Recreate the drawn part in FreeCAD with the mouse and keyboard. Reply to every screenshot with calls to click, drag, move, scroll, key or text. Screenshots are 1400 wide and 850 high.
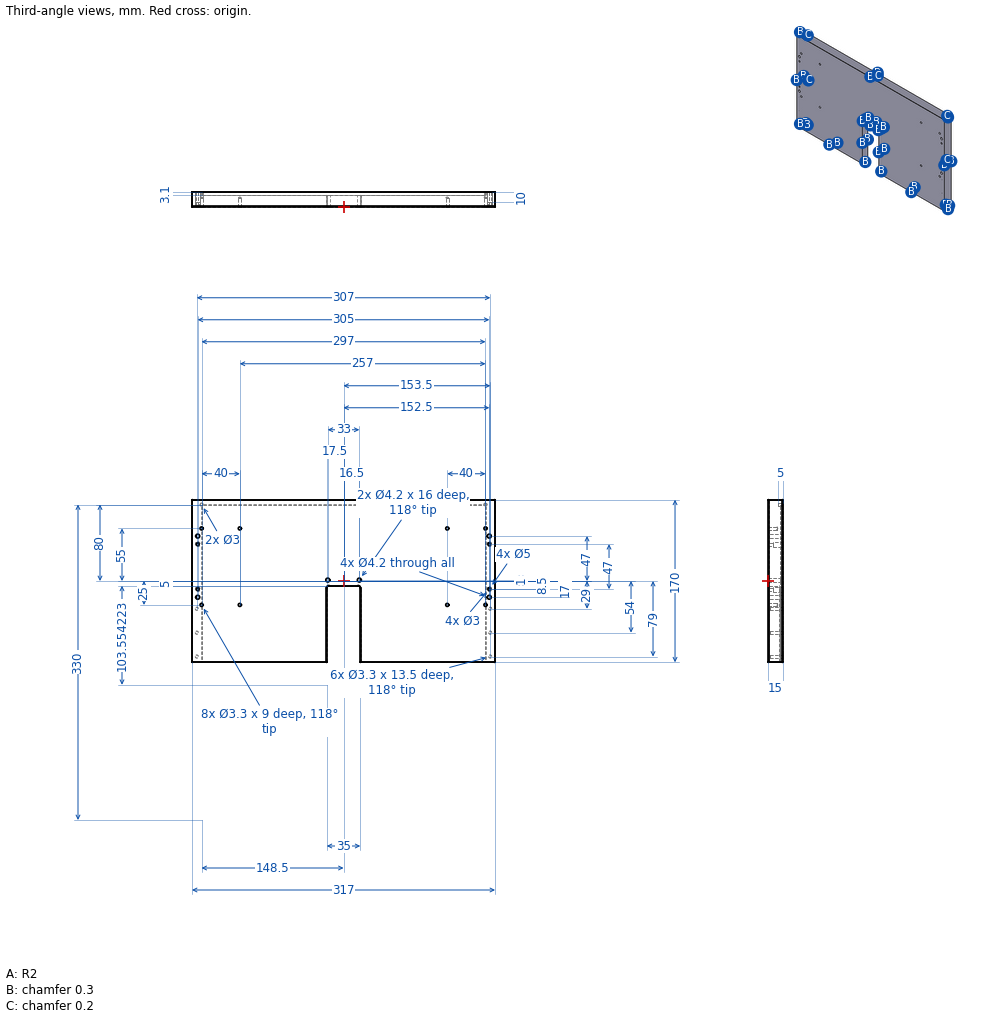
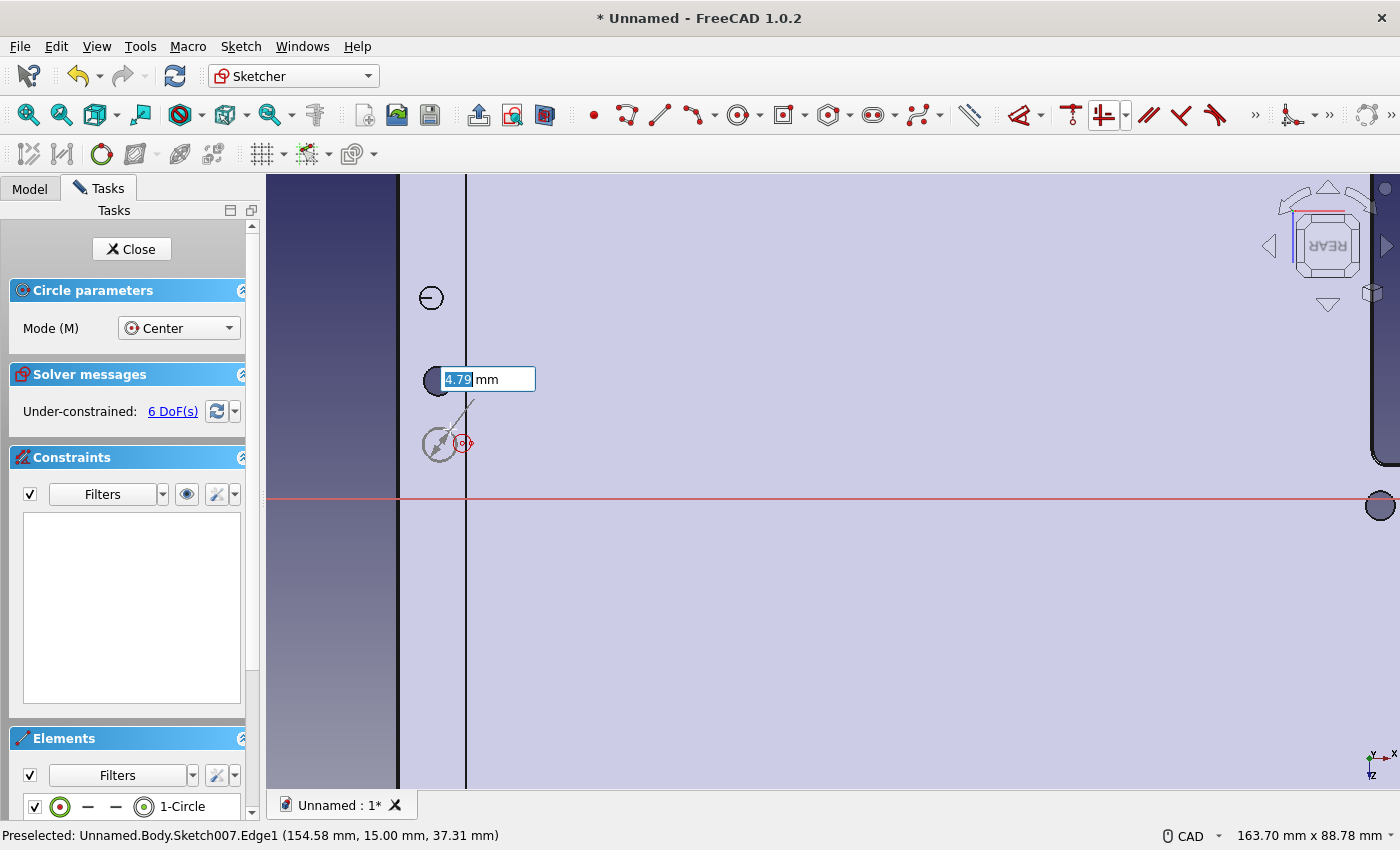
click(451, 428)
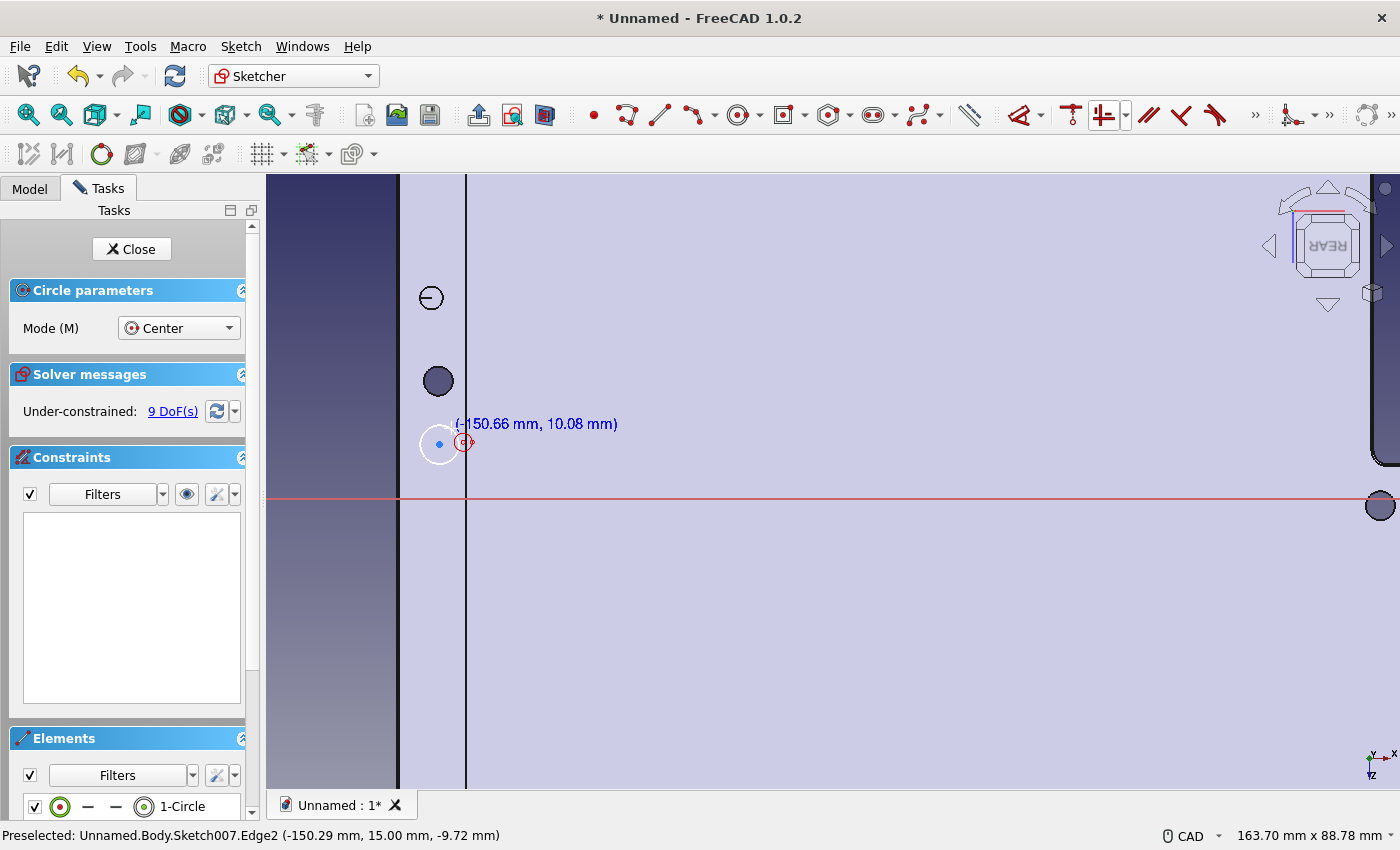
scroll(450, 429, down, 6)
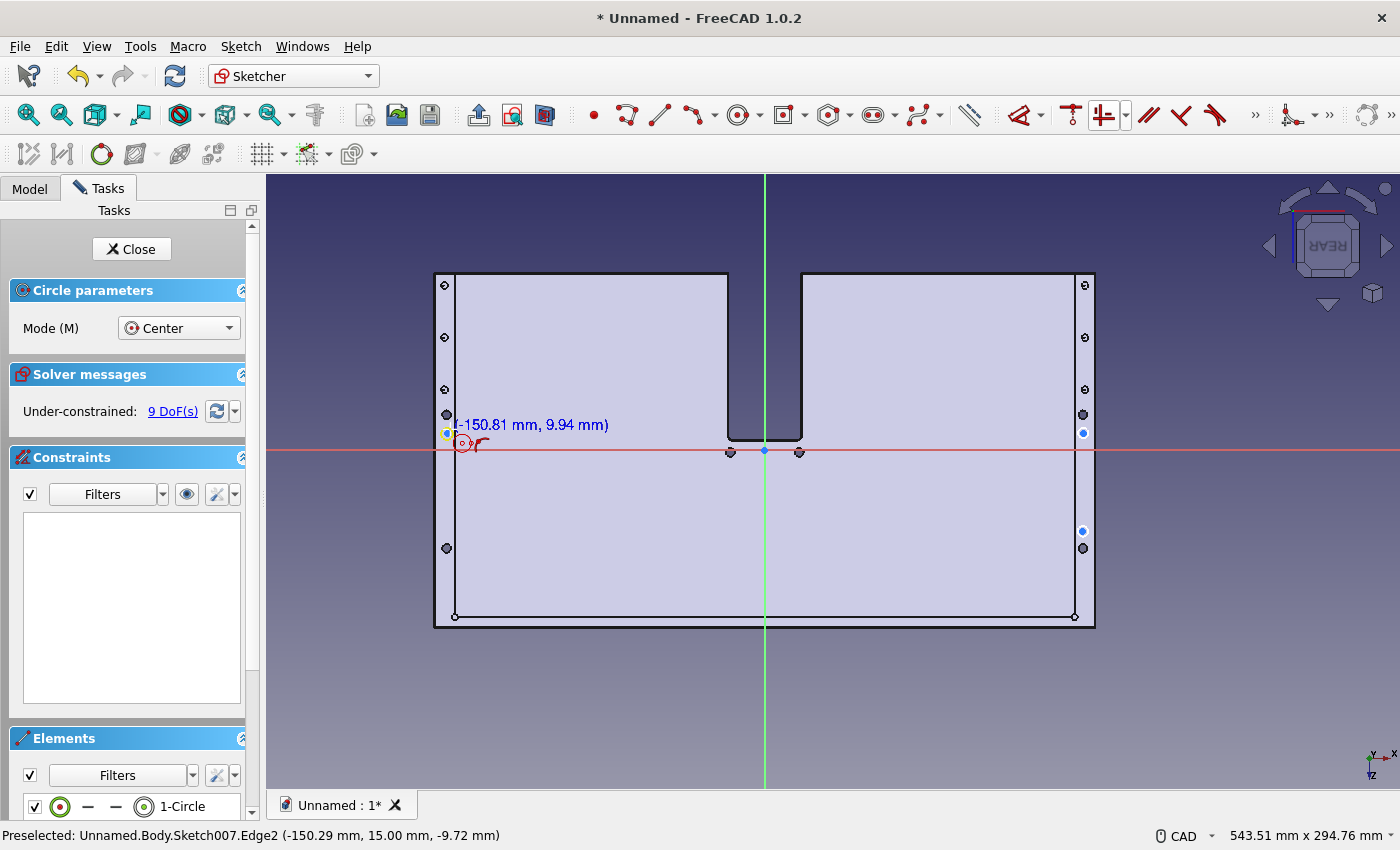
scroll(447, 531, up, 8)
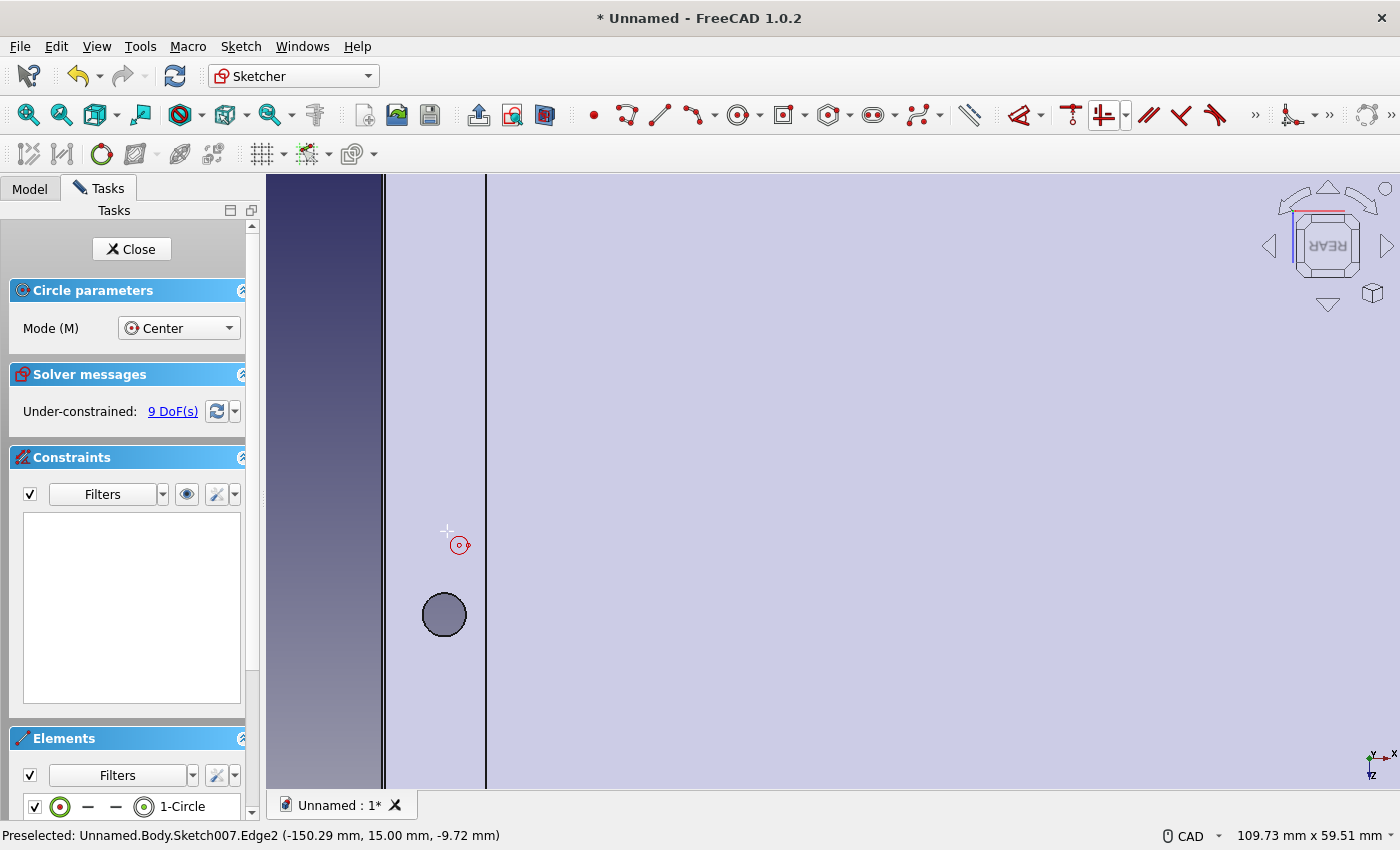
scroll(447, 531, down, 8)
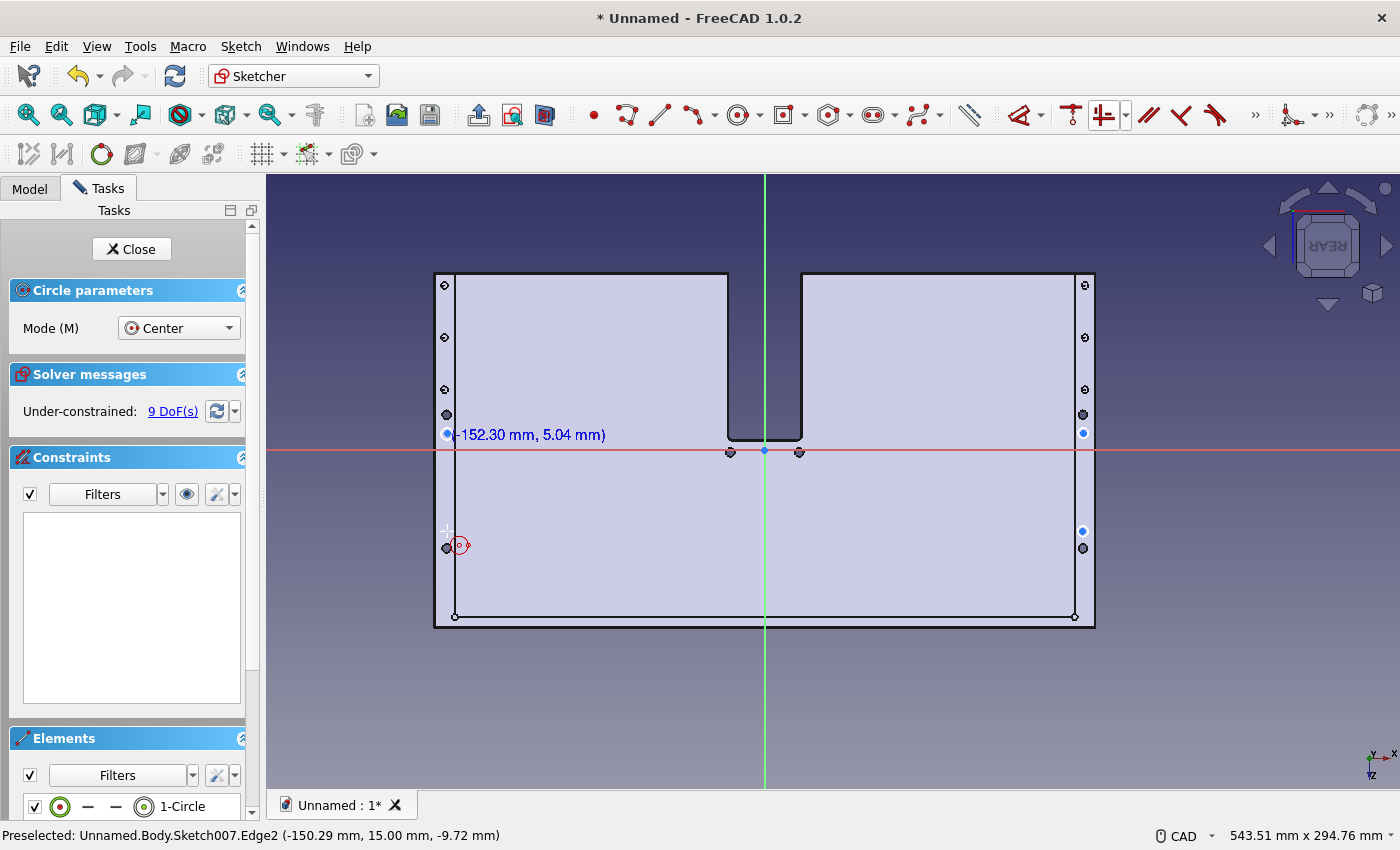
click(447, 531)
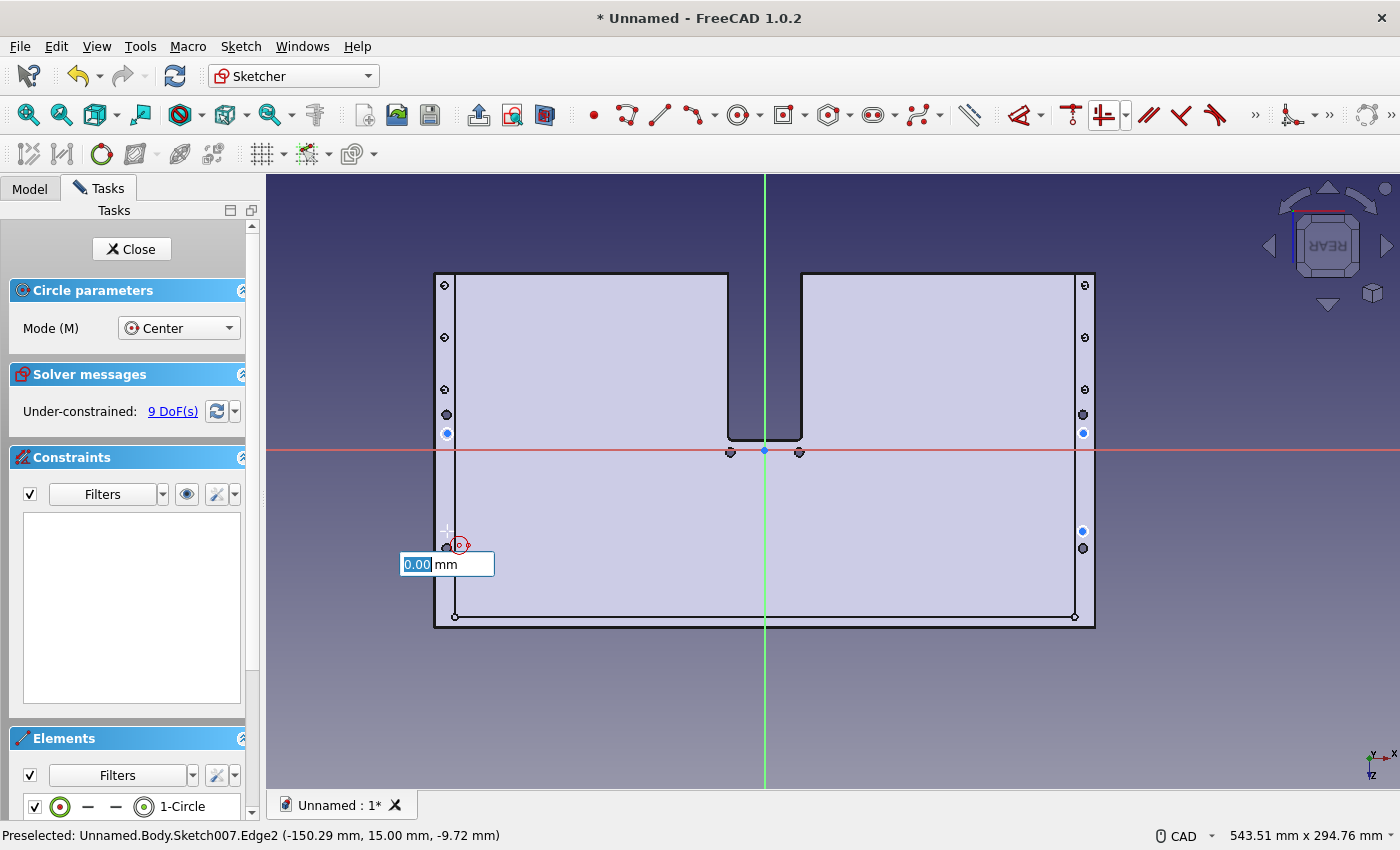
scroll(450, 527, up, 6)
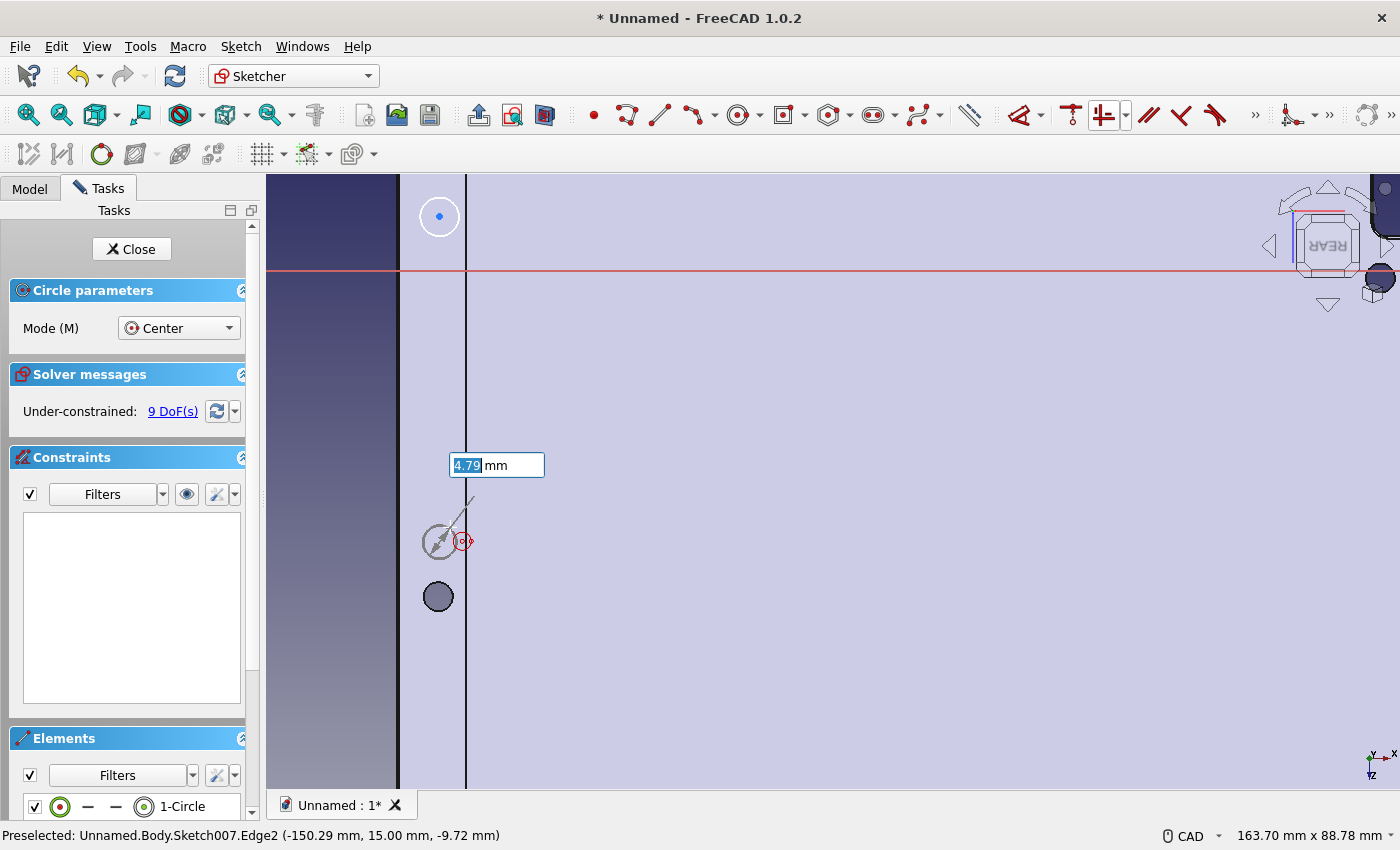
click(451, 526)
key(Escape)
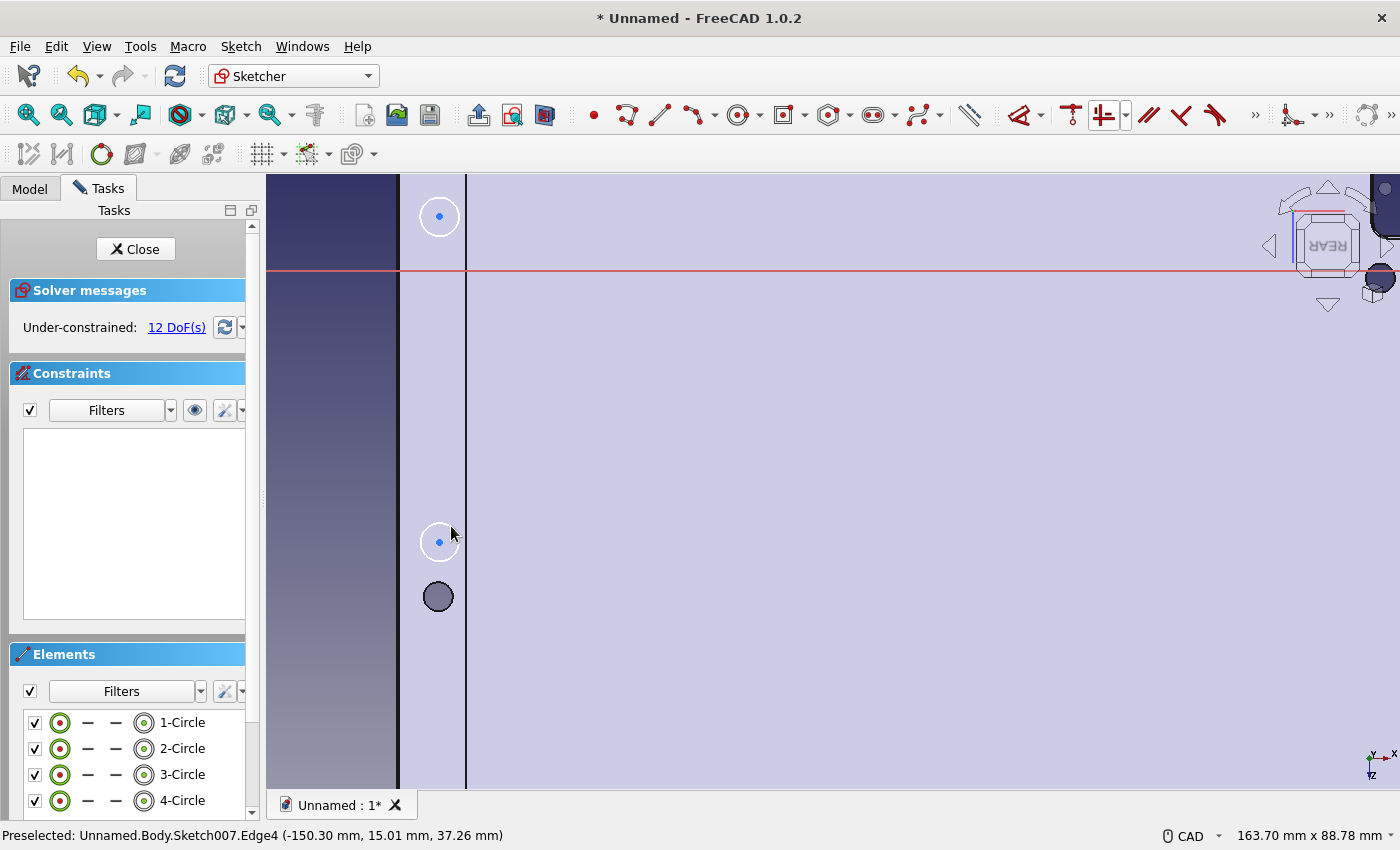
scroll(450, 527, down, 6)